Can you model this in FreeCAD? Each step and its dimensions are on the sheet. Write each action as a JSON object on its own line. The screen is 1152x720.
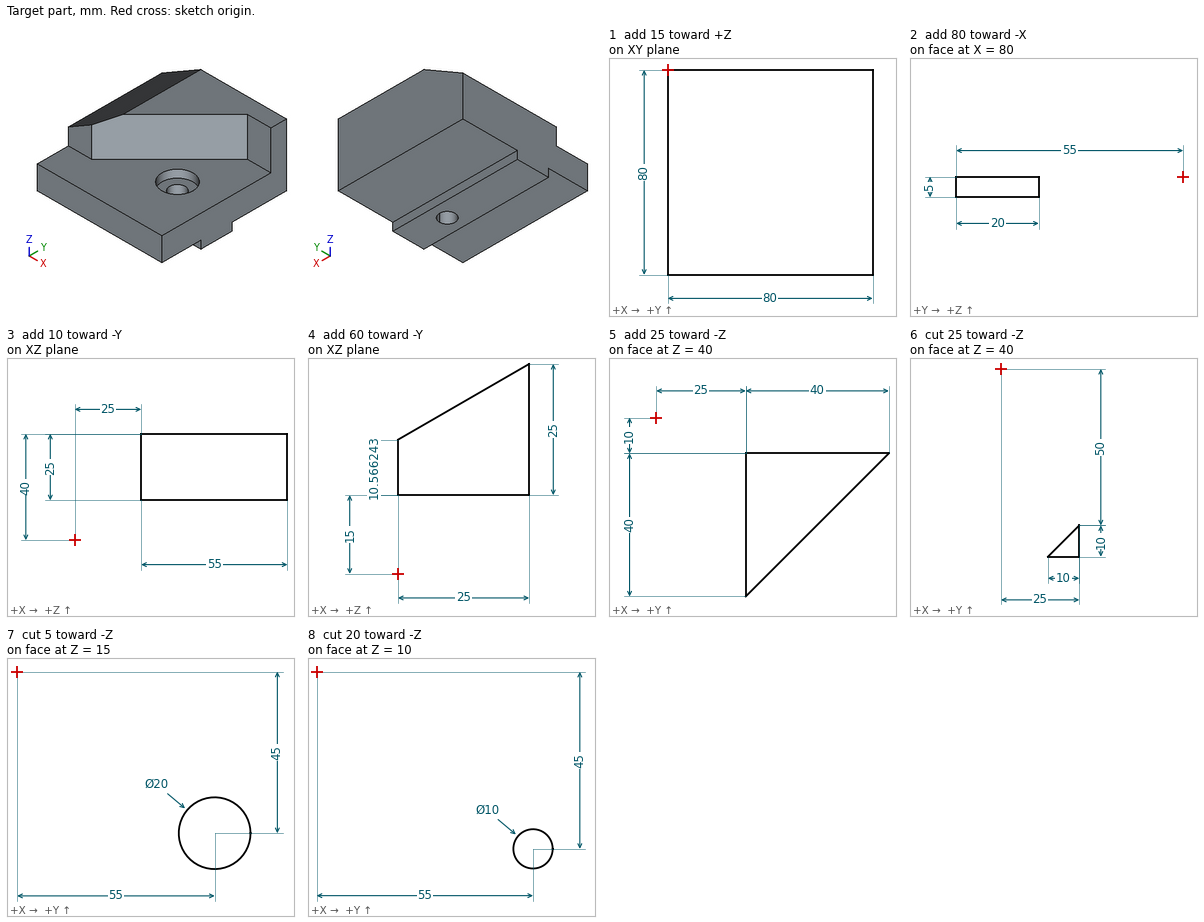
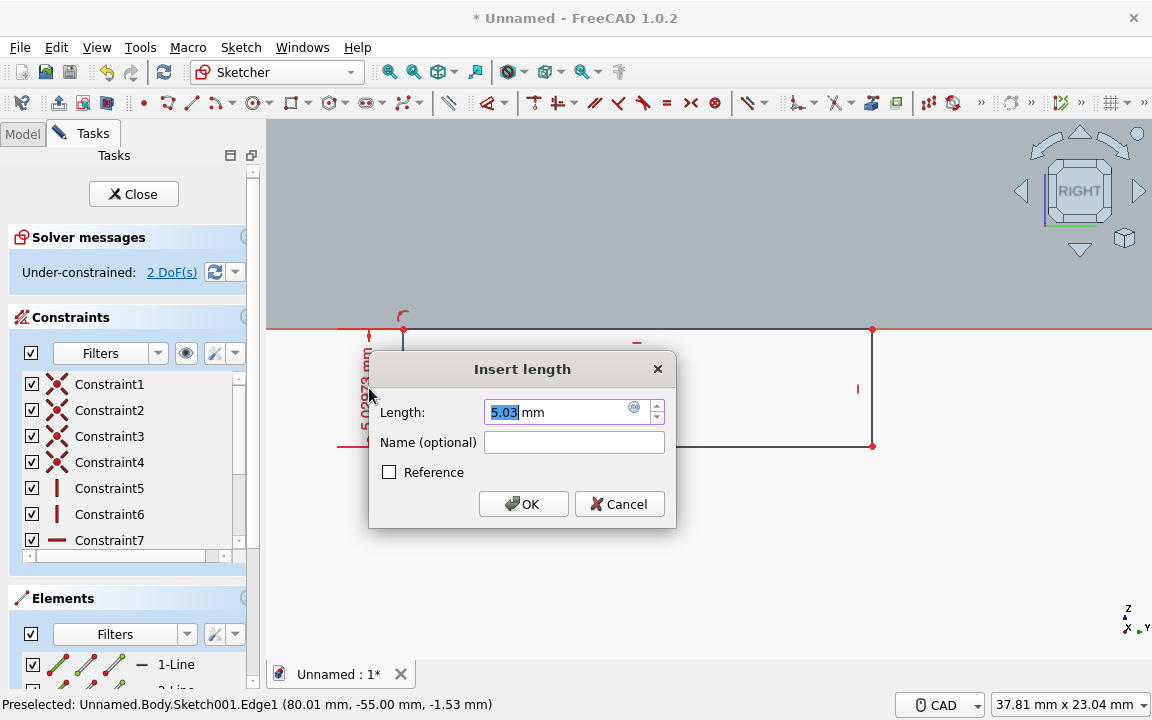
{"action": "type", "text": "5"}
{"action": "key", "text": "Return"}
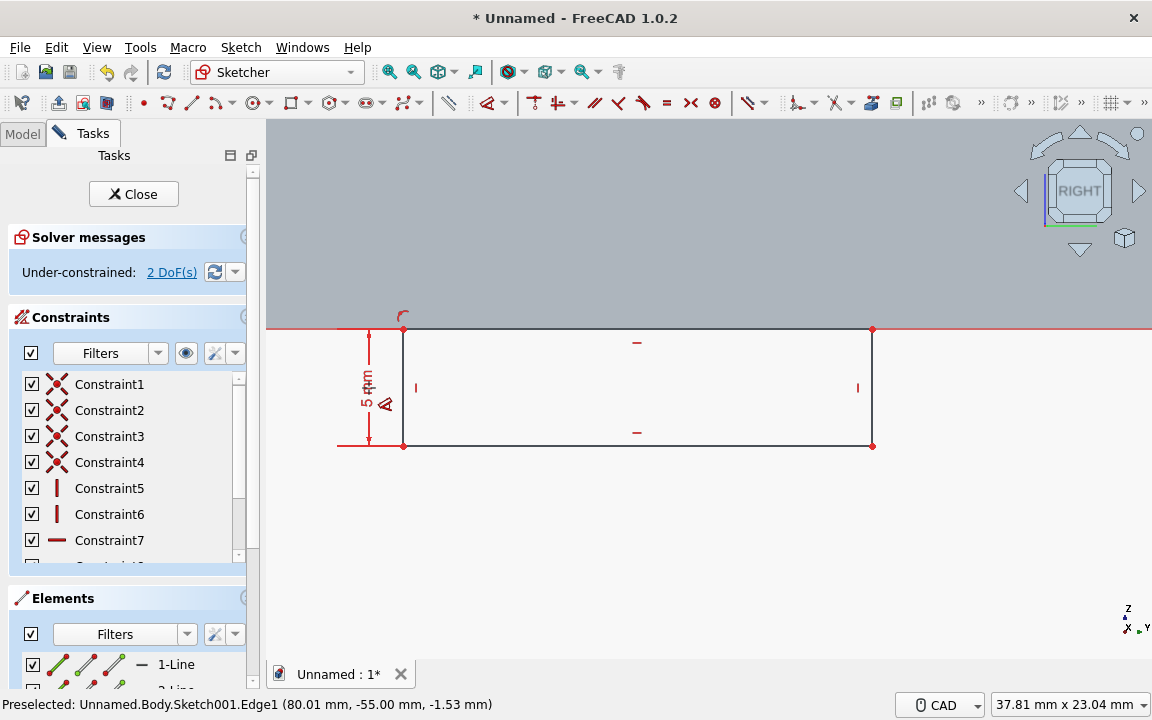
{"action": "left_click", "coordinate": [544, 446]}
{"action": "left_click", "coordinate": [637, 480]}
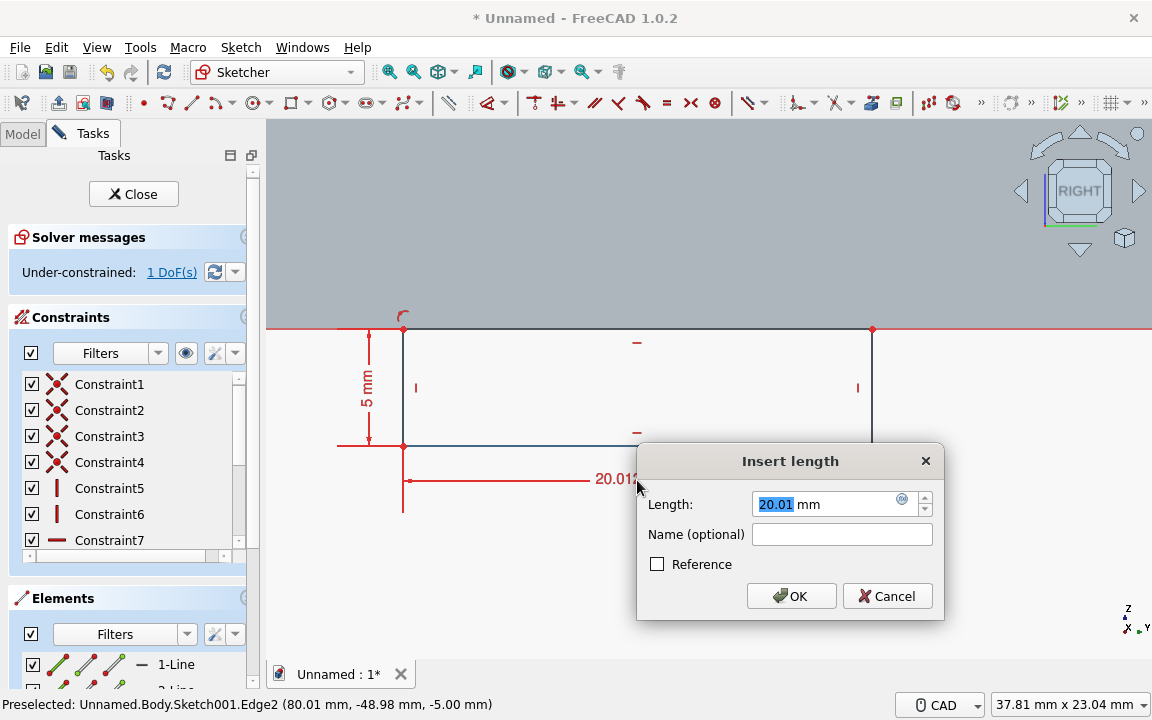
{"action": "type", "text": "20"}
{"action": "key", "text": "Return"}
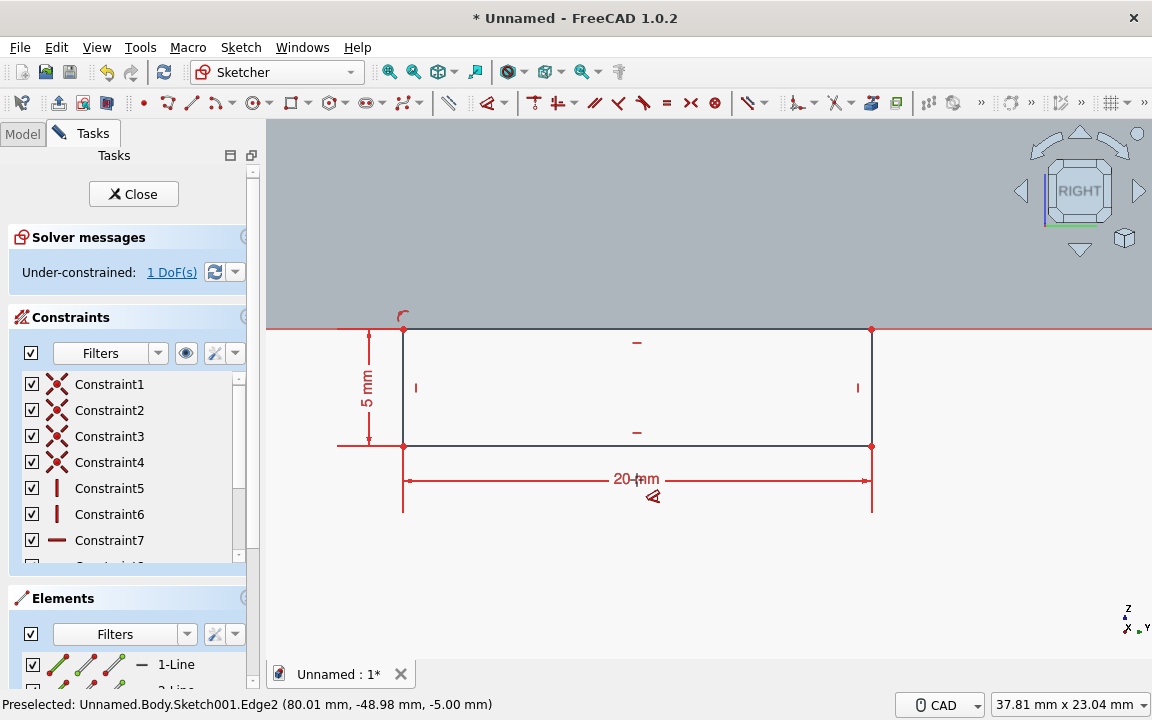
{"action": "left_click", "coordinate": [403, 329]}
{"action": "left_click", "coordinate": [695, 295]}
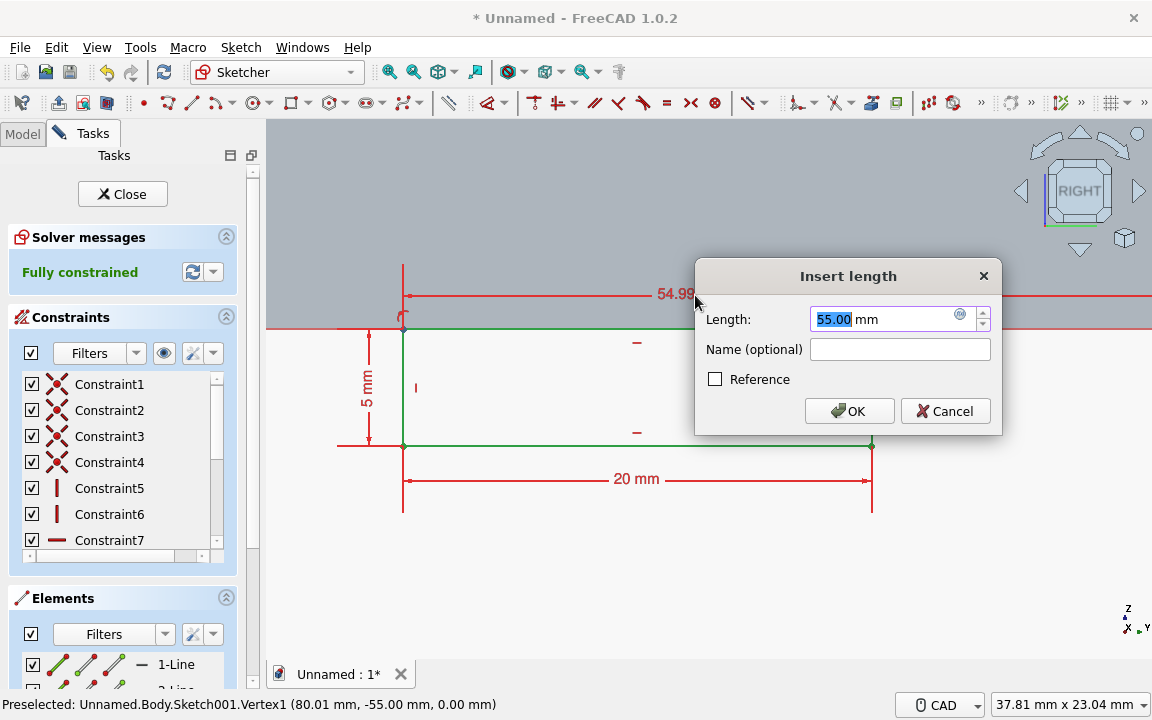
{"action": "type", "text": "55"}
{"action": "key", "text": "Return"}
{"action": "key", "text": "Escape"}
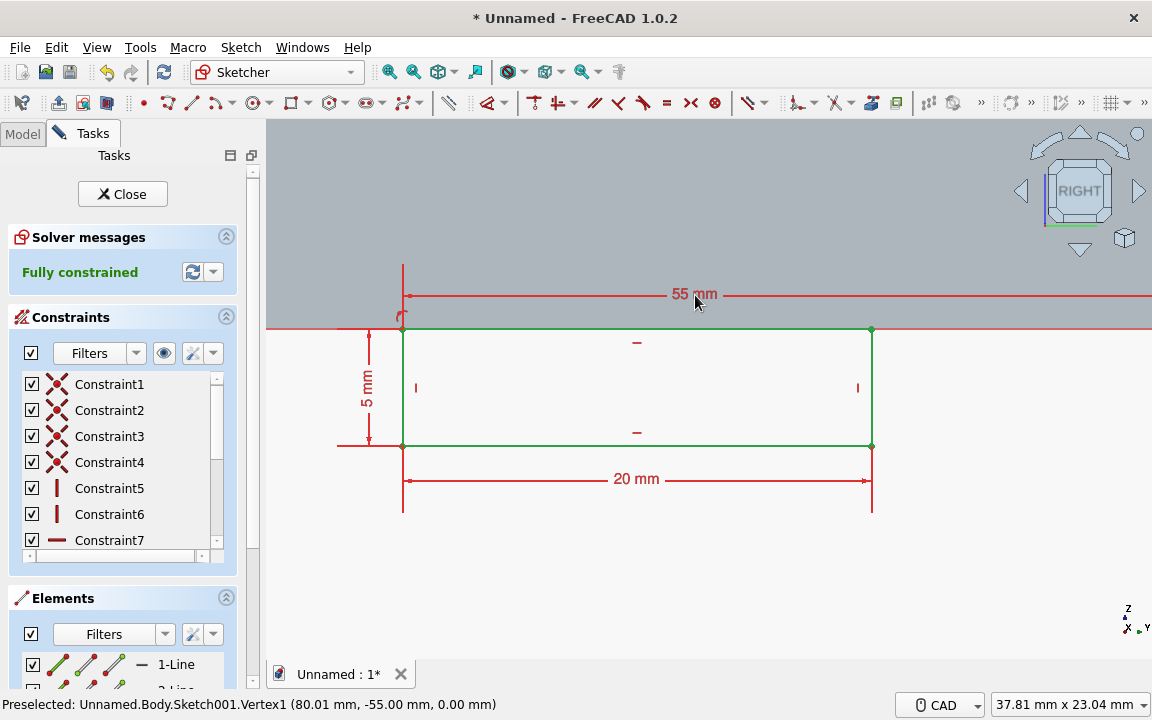
{"action": "left_click", "coordinate": [123, 194]}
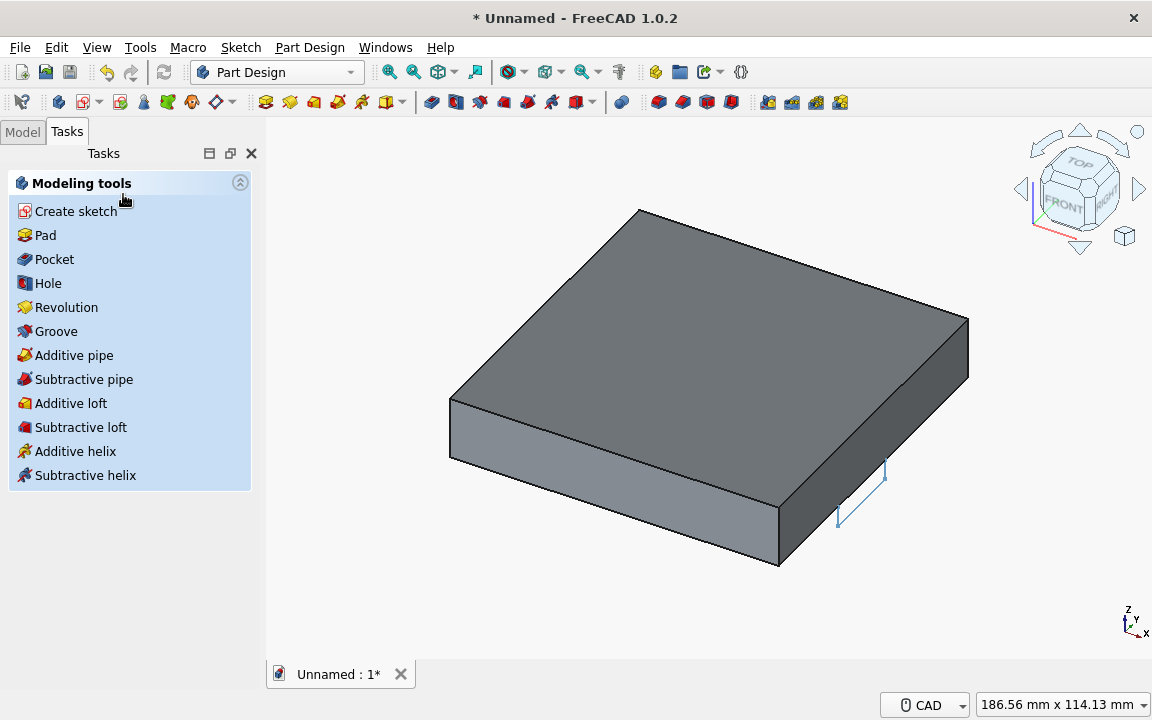
{"action": "left_click", "coordinate": [266, 102]}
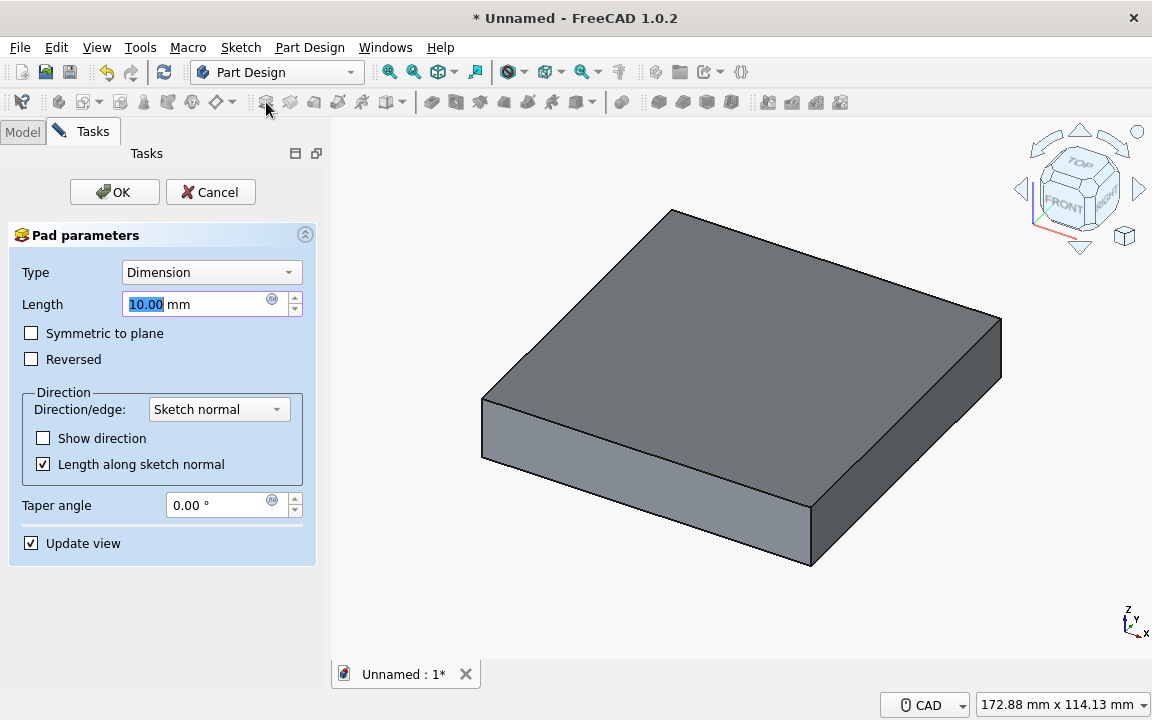
{"action": "type", "text": "80"}
{"action": "key", "text": "Tab"}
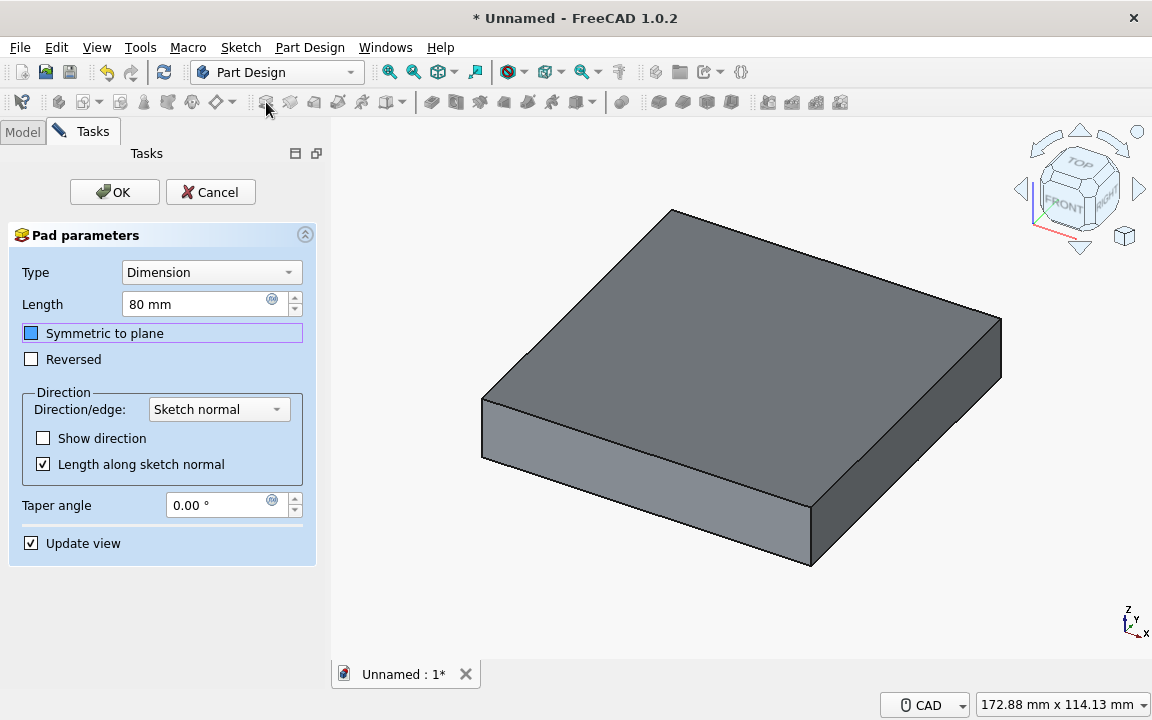
{"action": "left_click", "coordinate": [30, 359]}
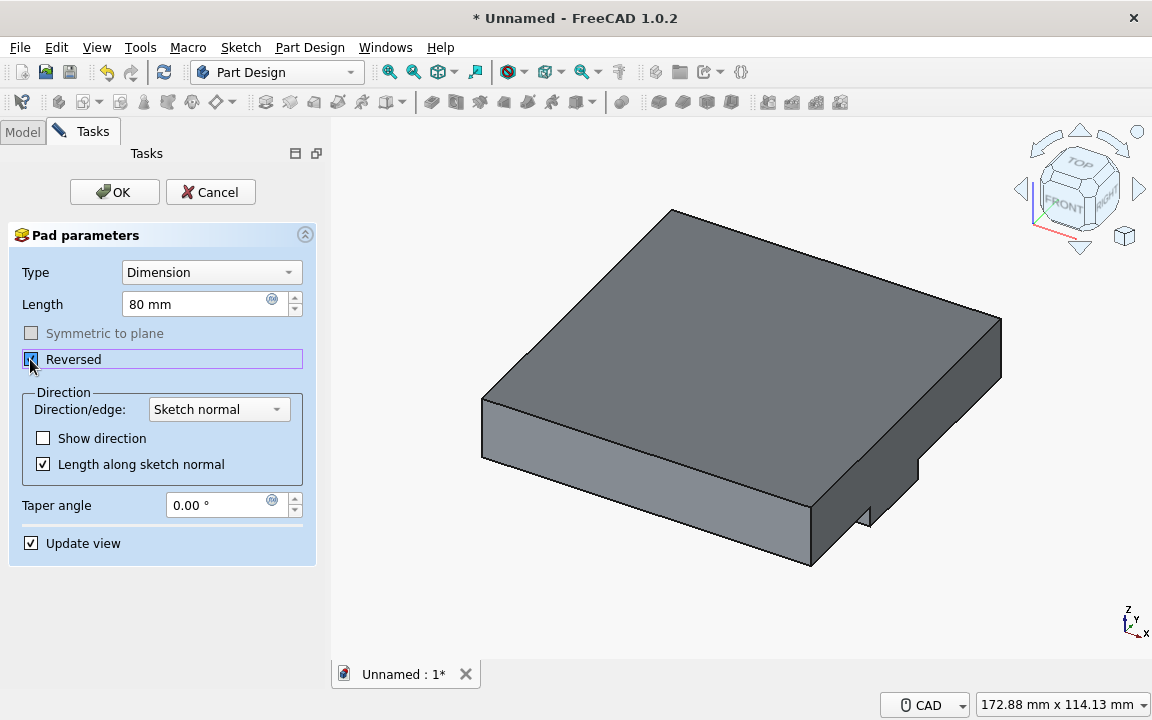
{"action": "left_click", "coordinate": [115, 192]}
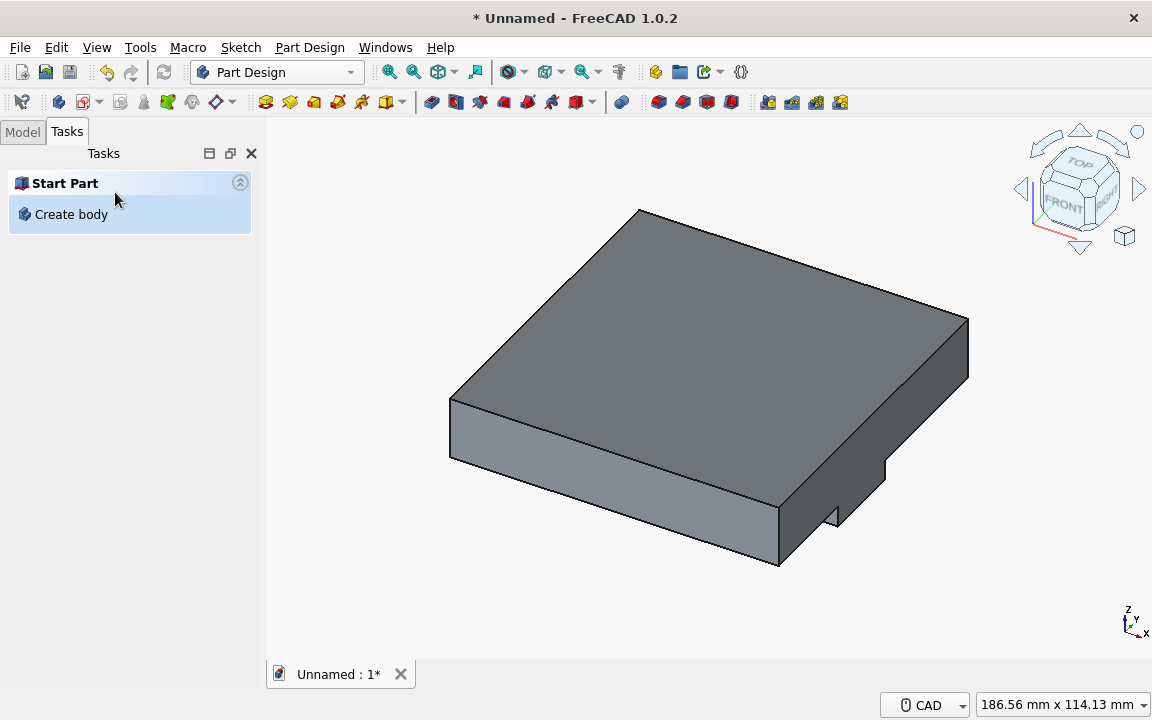
{"action": "left_click", "coordinate": [84, 102]}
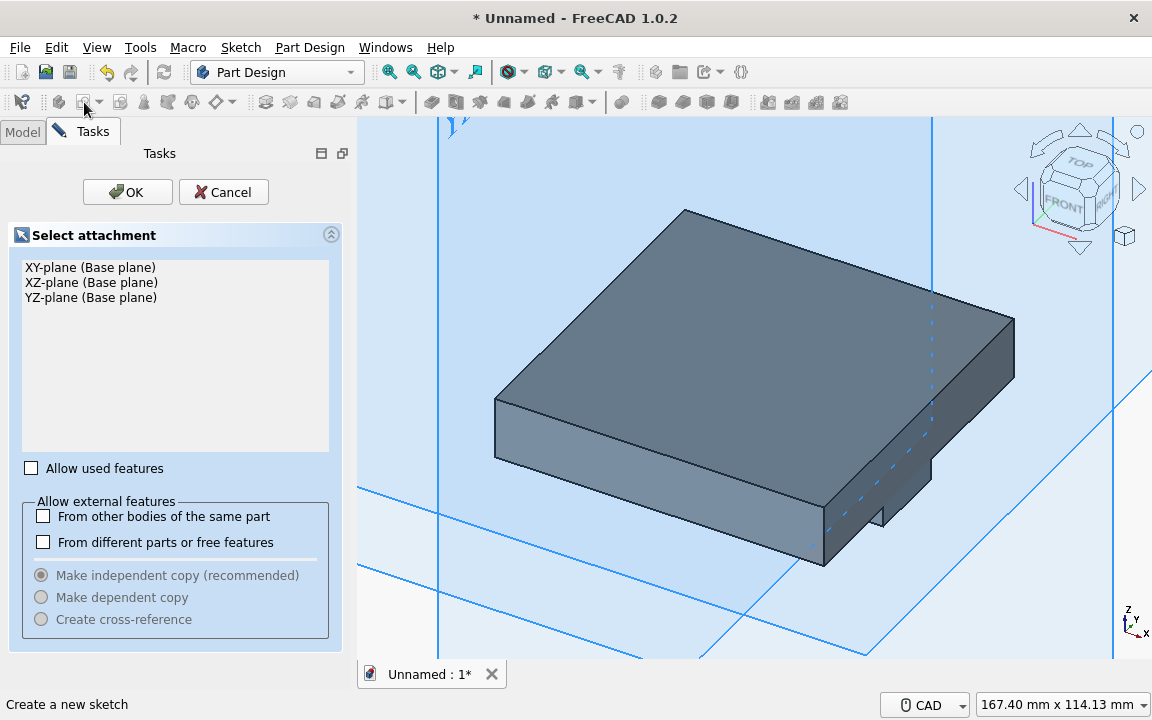
{"action": "left_click", "coordinate": [82, 282]}